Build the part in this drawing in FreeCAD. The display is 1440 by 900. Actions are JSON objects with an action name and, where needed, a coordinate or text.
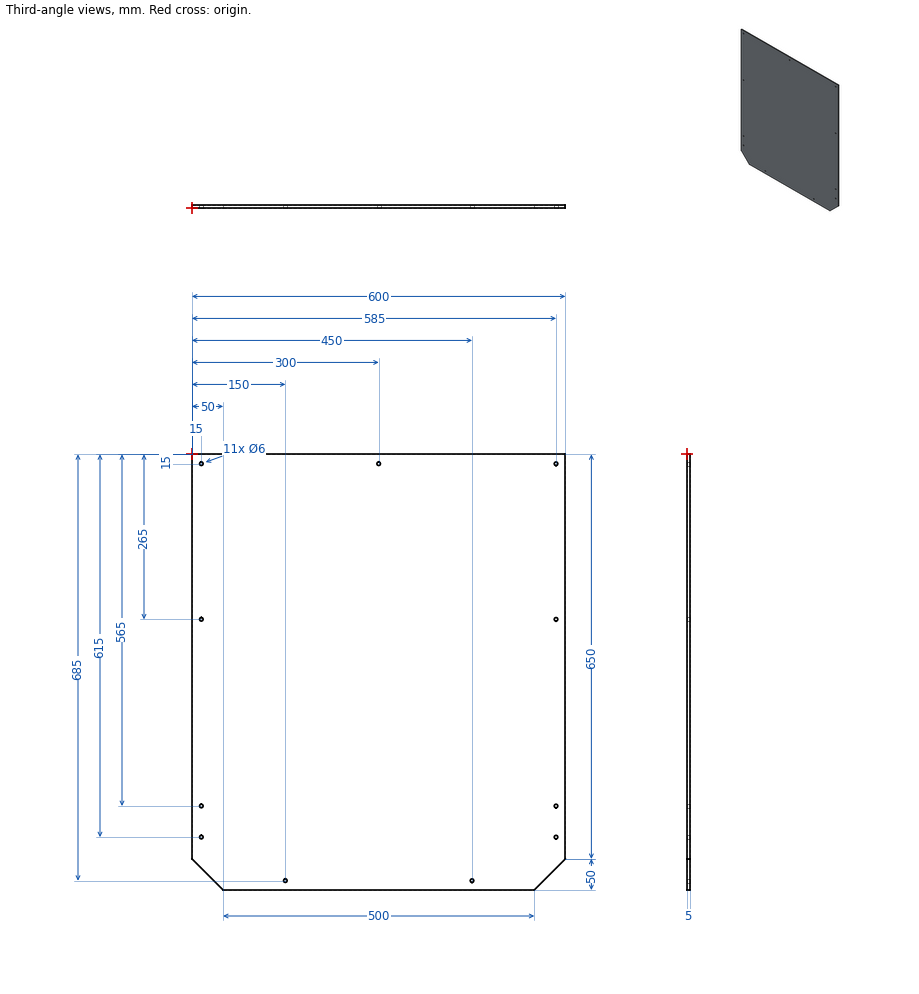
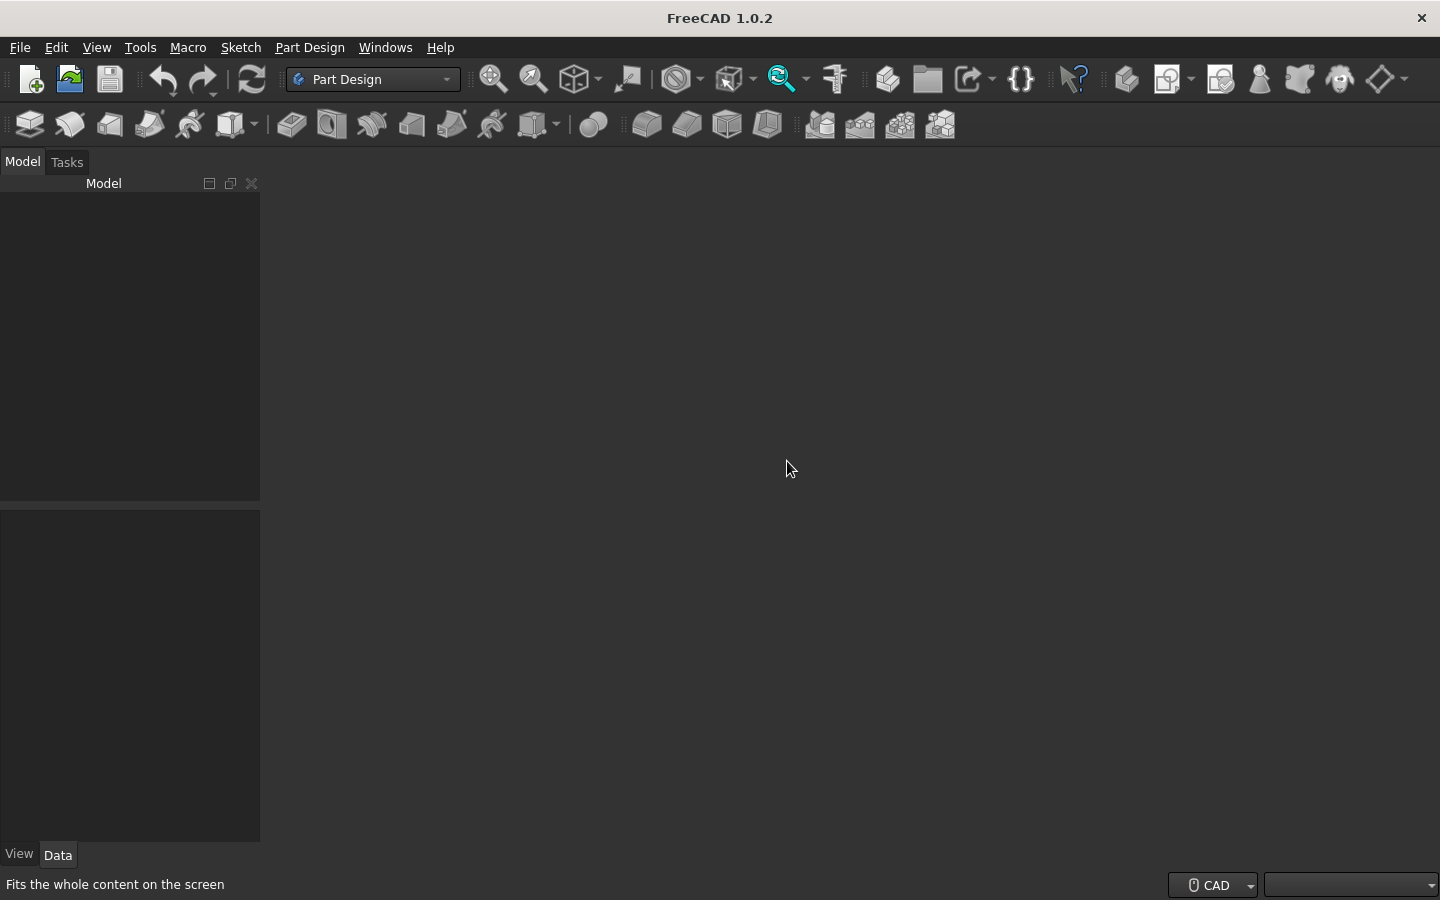
{"action": "key", "text": "ctrl+n"}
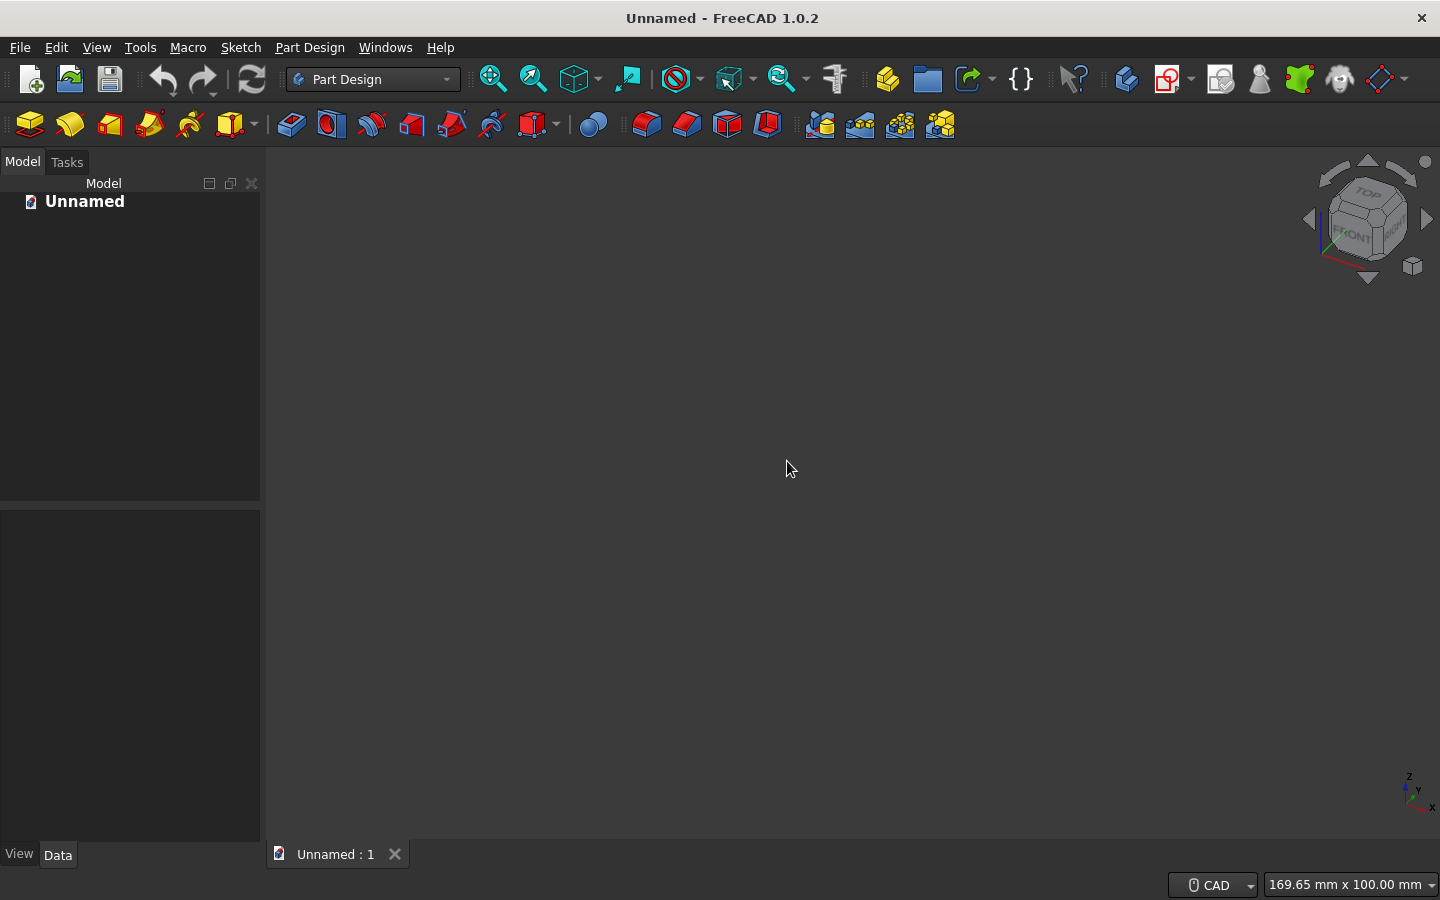
{"action": "left_click", "coordinate": [1168, 80]}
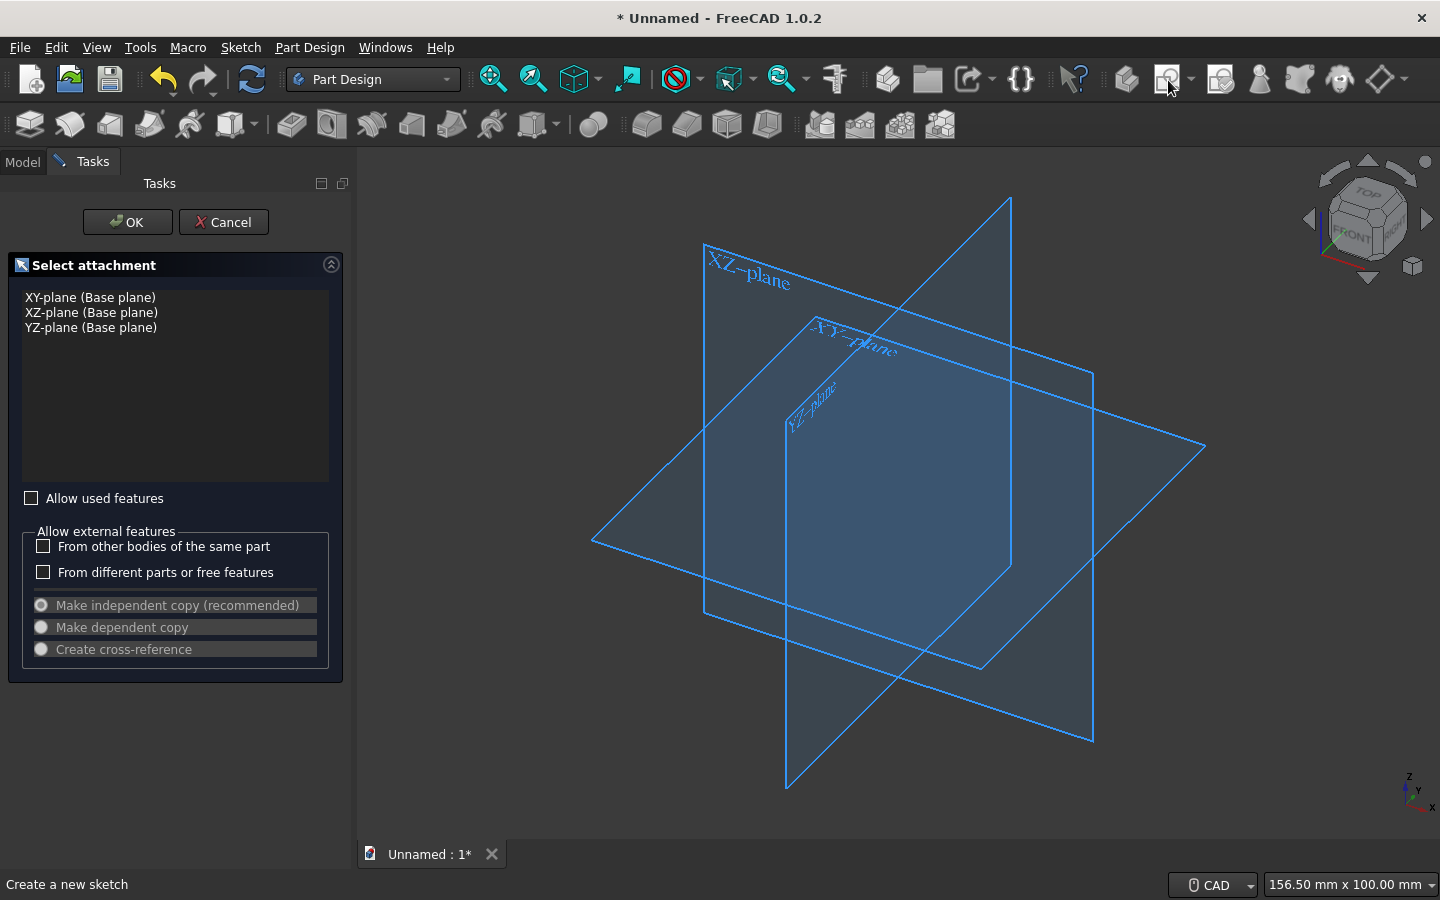
{"action": "left_click", "coordinate": [82, 312]}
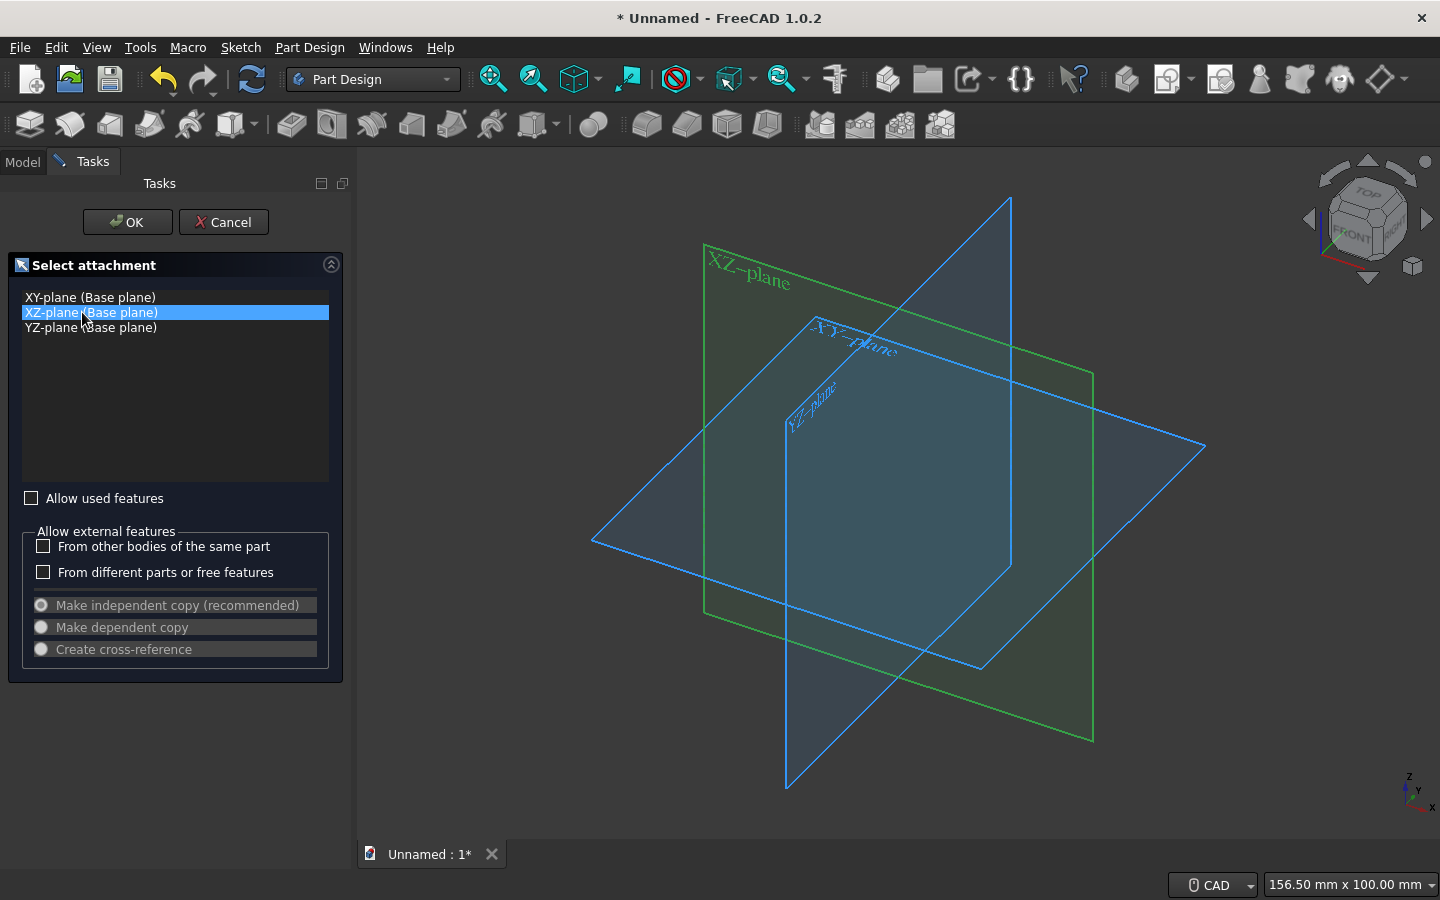
{"action": "left_click", "coordinate": [128, 222]}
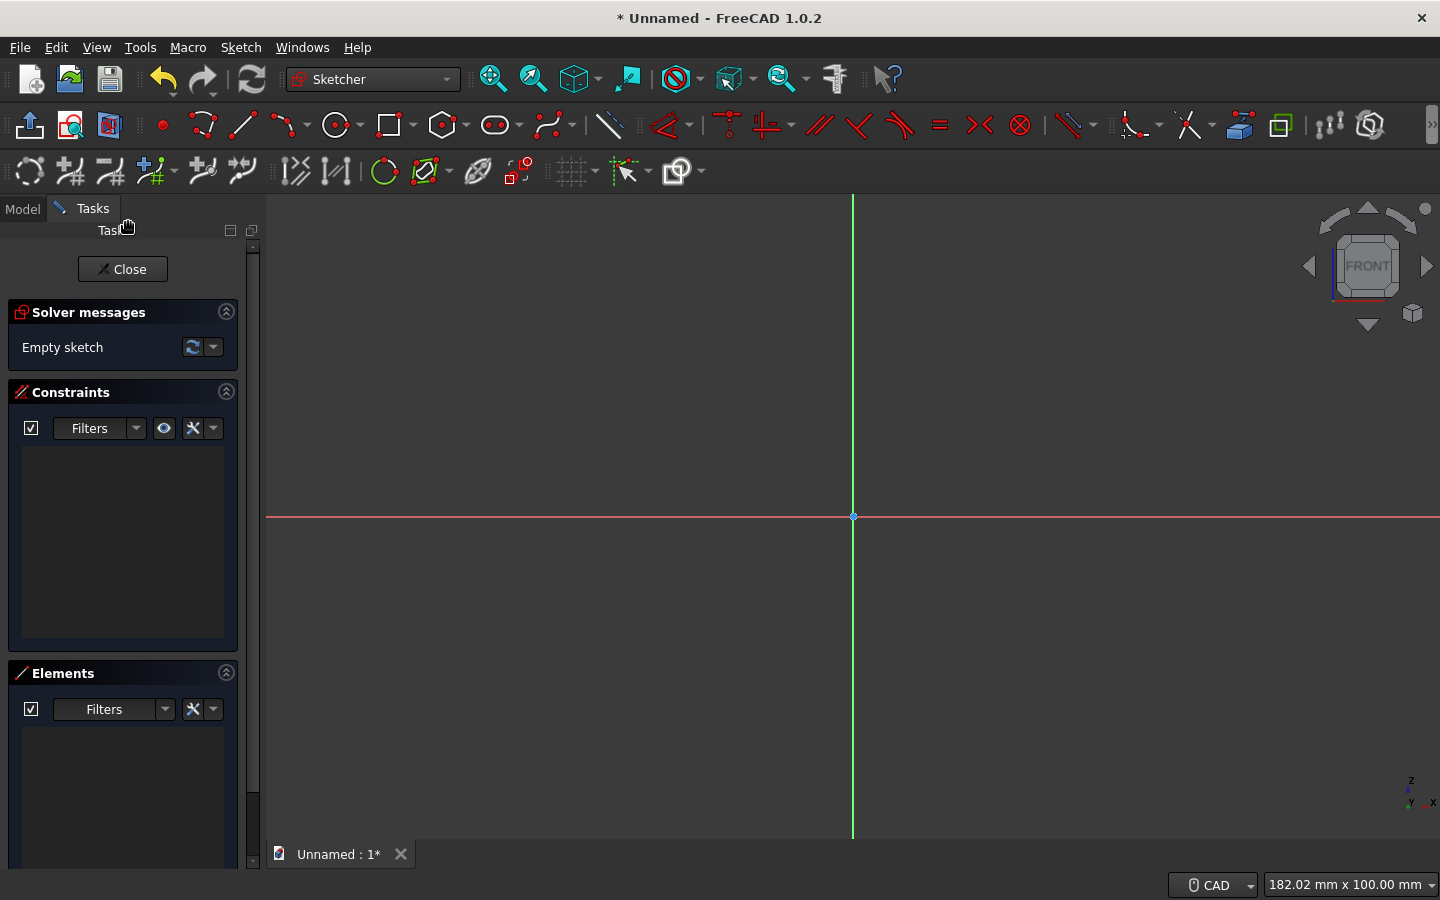
{"action": "scroll", "coordinate": [585, 291], "scroll_direction": "down", "scroll_amount": 12}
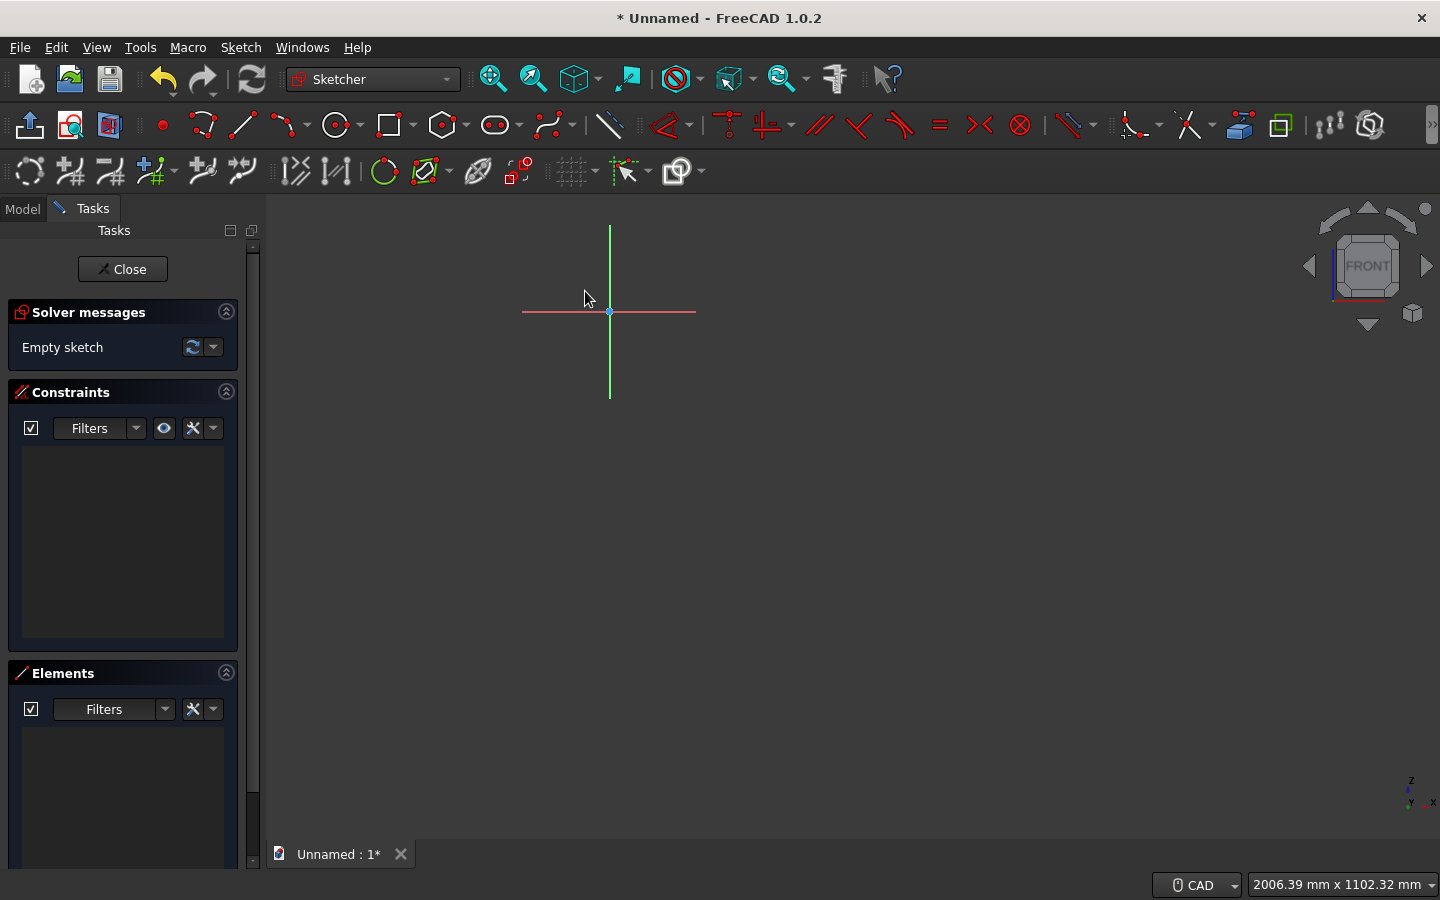
{"action": "key", "text": "g m"}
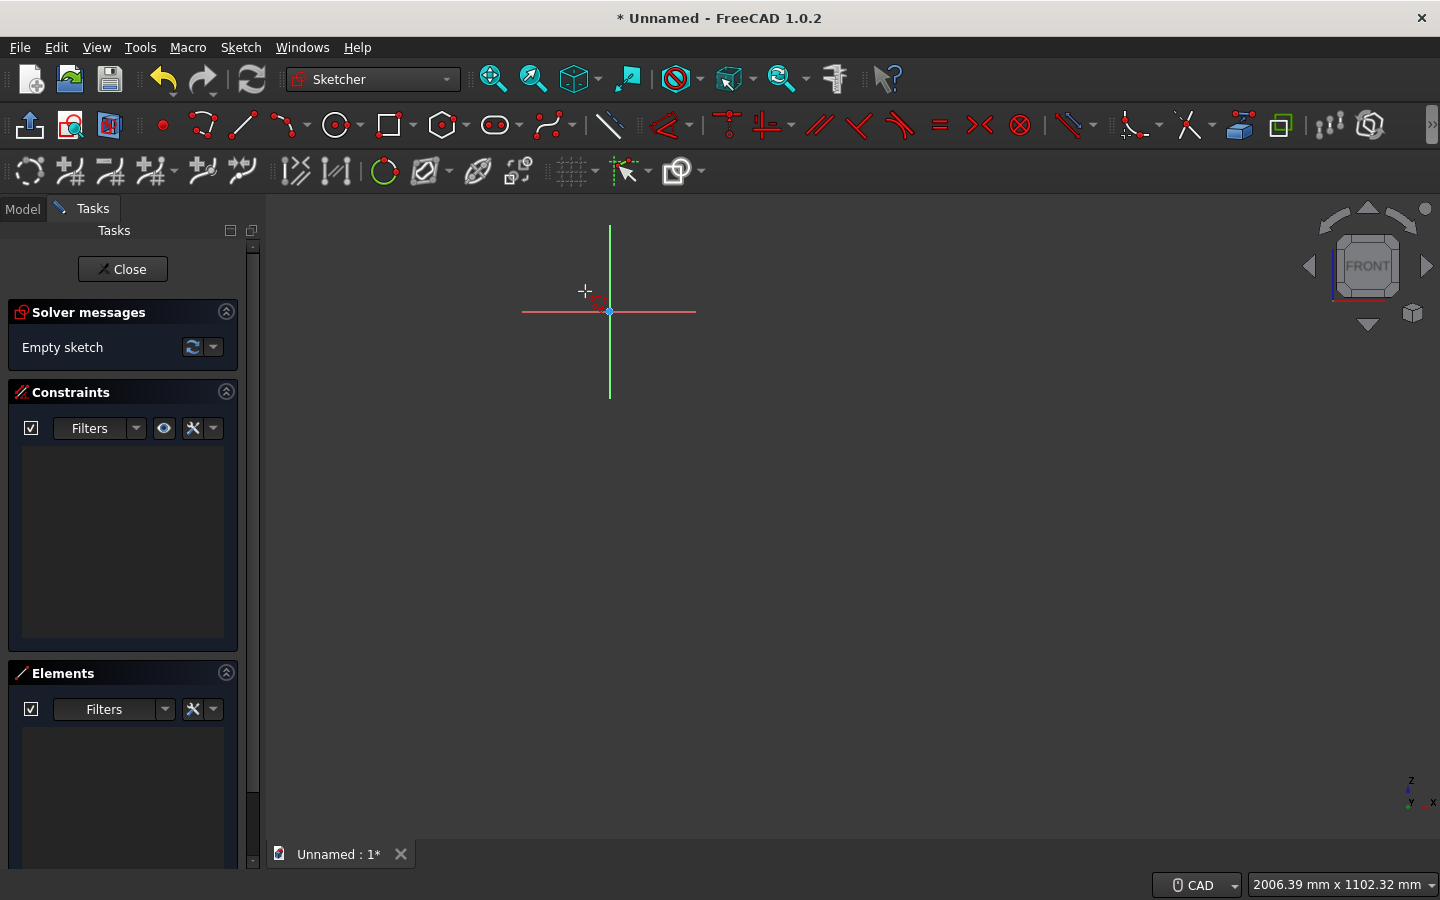
{"action": "left_click", "coordinate": [610, 312]}
{"action": "left_click", "coordinate": [961, 321]}
{"action": "left_click", "coordinate": [961, 692]}
{"action": "left_click", "coordinate": [931, 721]}
{"action": "left_click", "coordinate": [639, 721]}
{"action": "left_click", "coordinate": [619, 692]}
{"action": "left_click", "coordinate": [610, 312]}
{"action": "key", "text": "Escape"}
{"action": "key", "text": "Escape"}